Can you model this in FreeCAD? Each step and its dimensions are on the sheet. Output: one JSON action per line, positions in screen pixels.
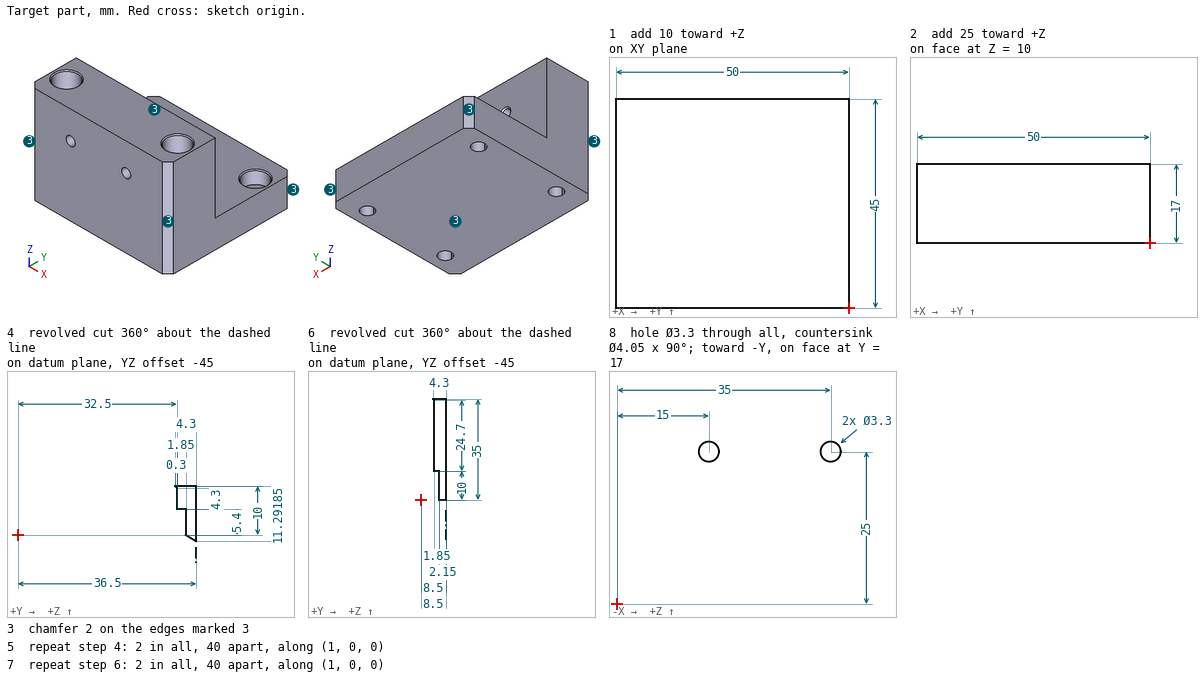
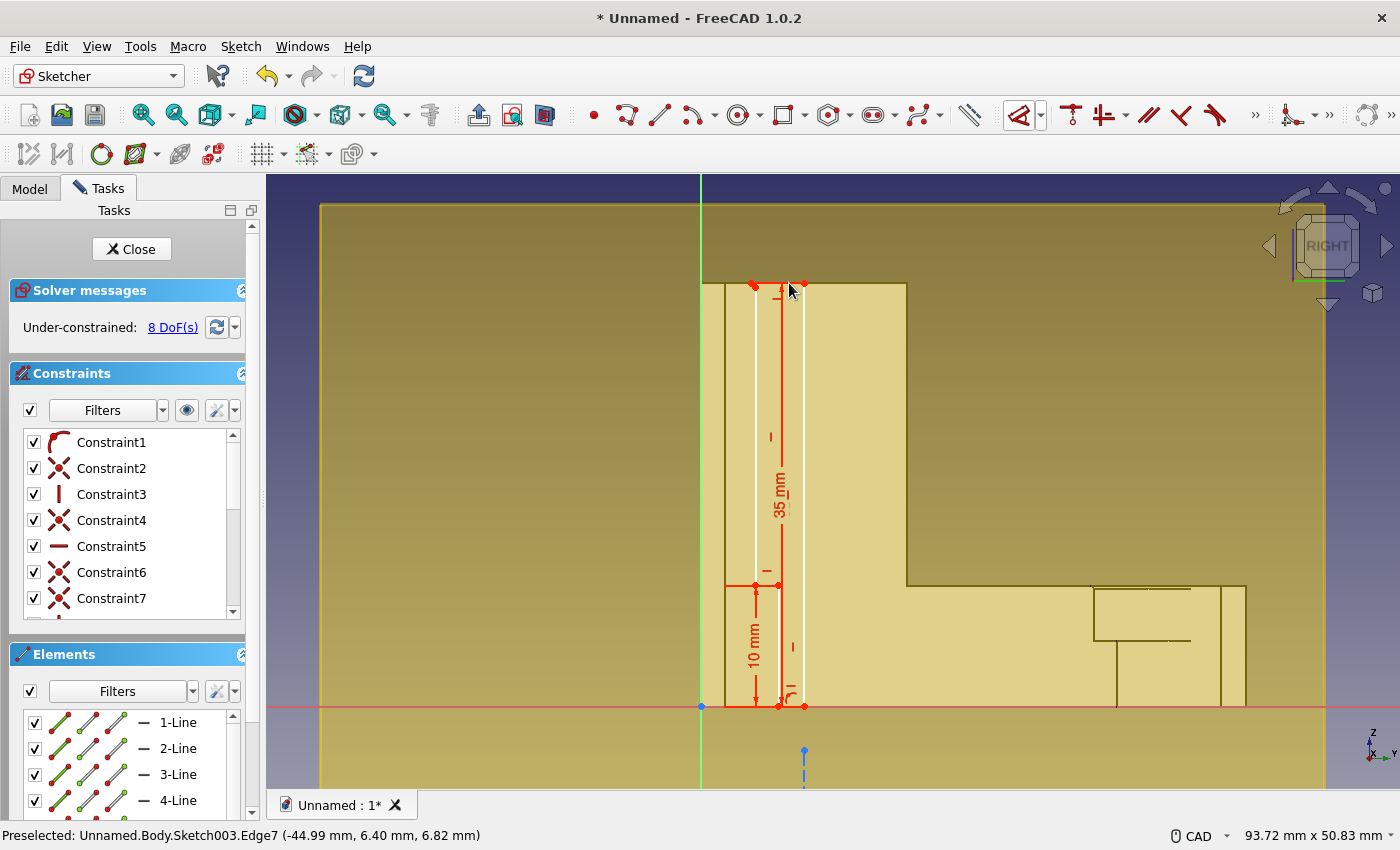
{"action": "left_click", "coordinate": [788, 283]}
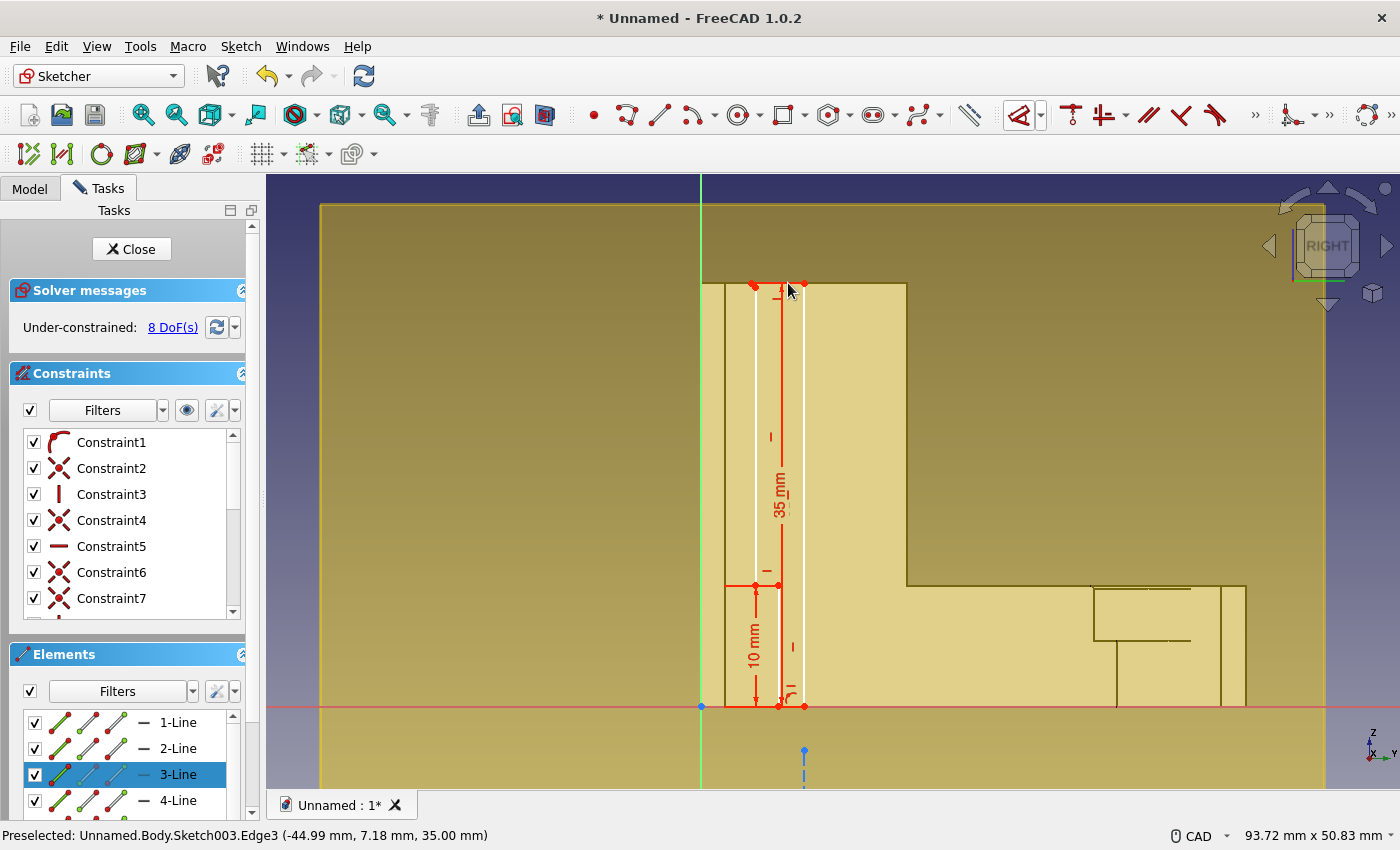
{"action": "key", "text": "l"}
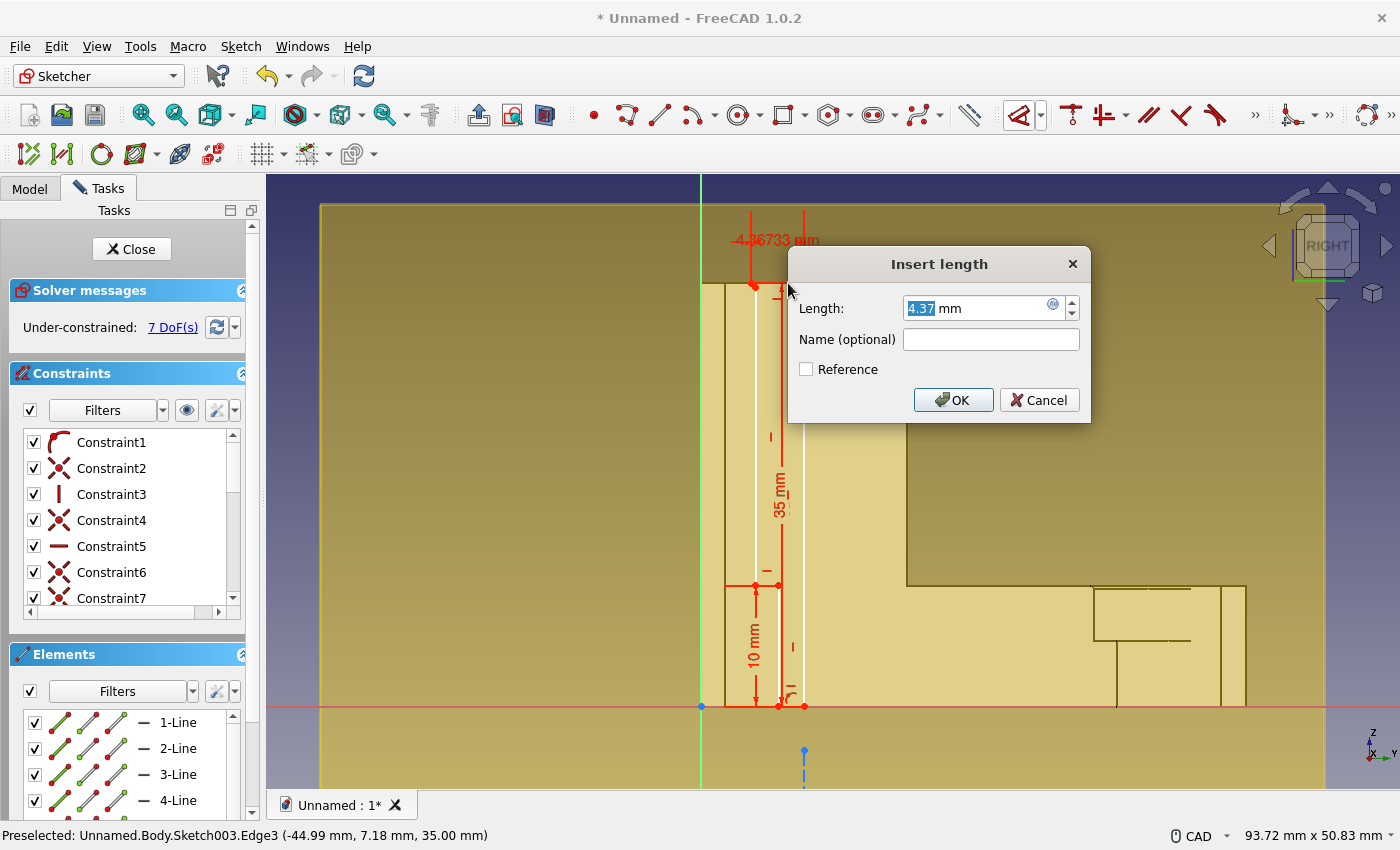
{"action": "type", "text": "4.3"}
{"action": "key", "text": "Return"}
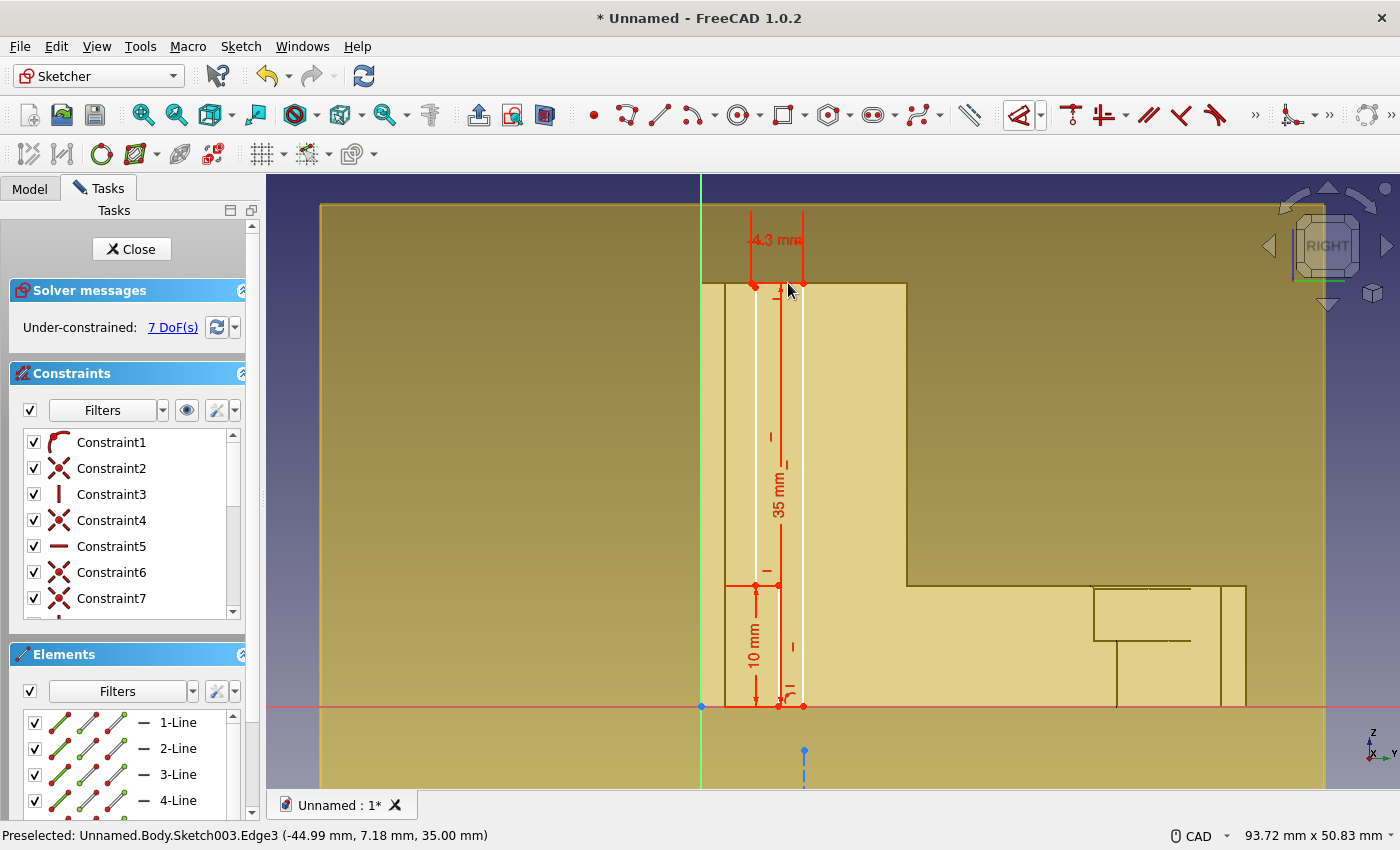
{"action": "scroll", "coordinate": [788, 707], "scroll_direction": "up", "scroll_amount": 3}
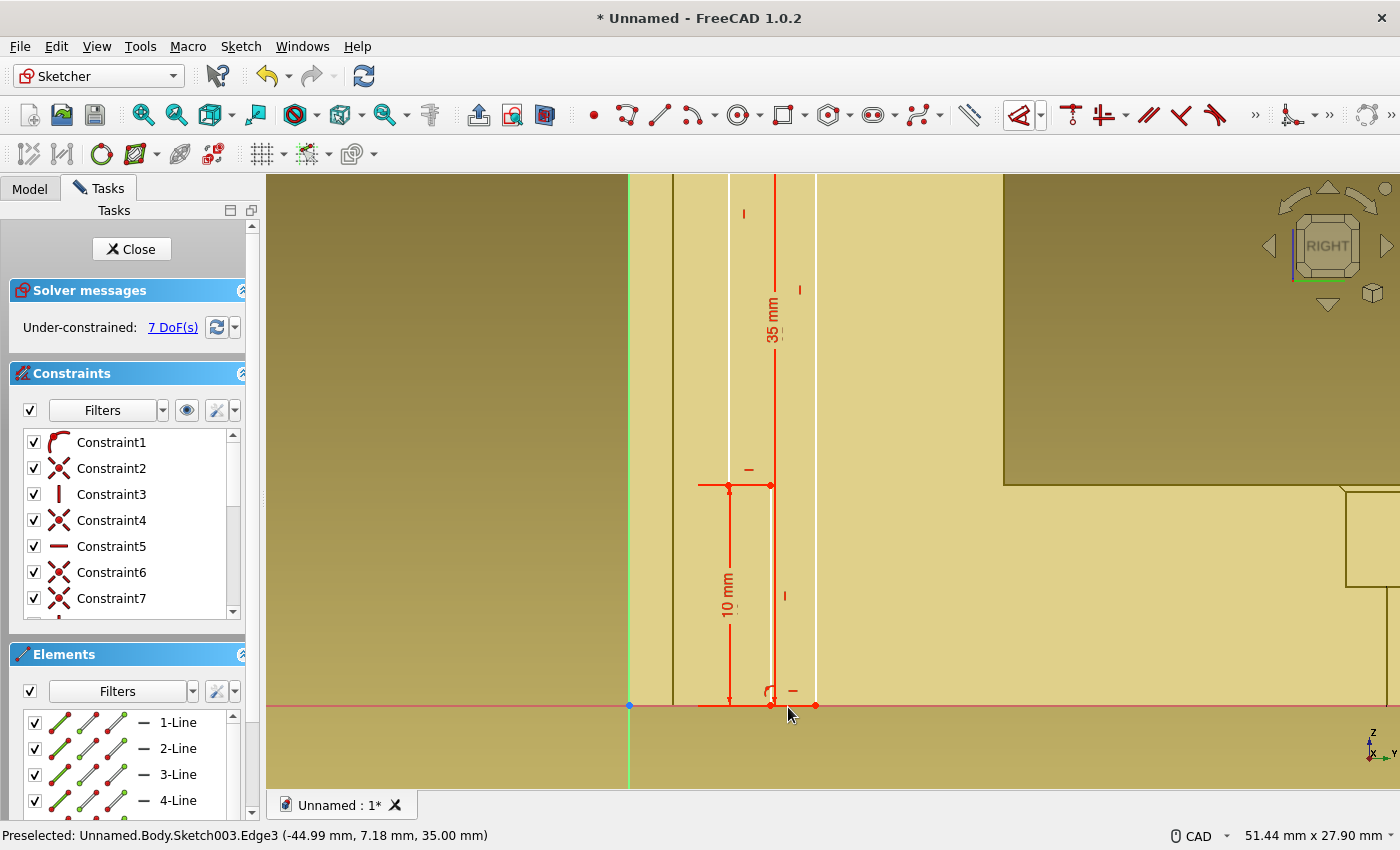
{"action": "left_click", "coordinate": [789, 706]}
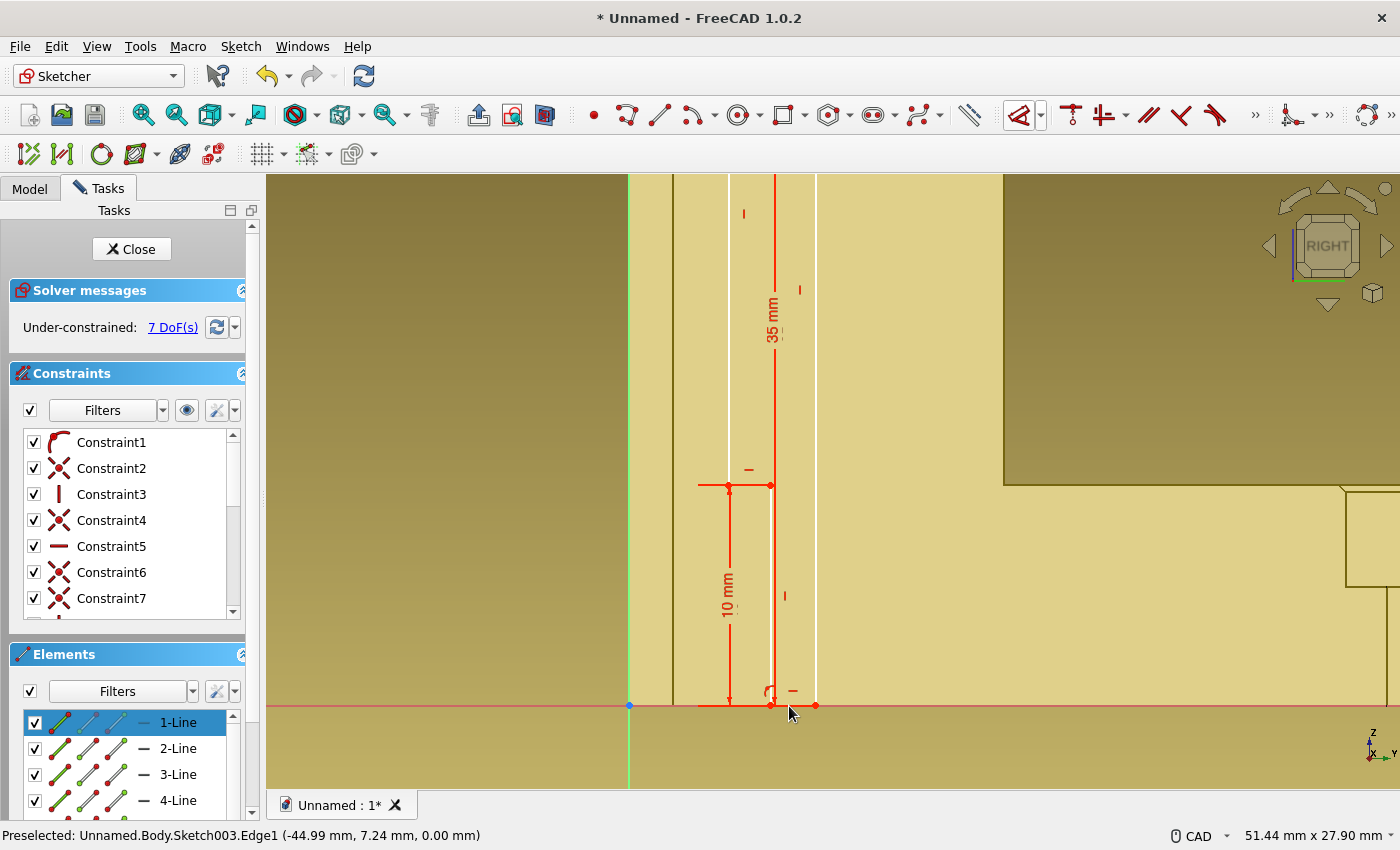
{"action": "key", "text": "l"}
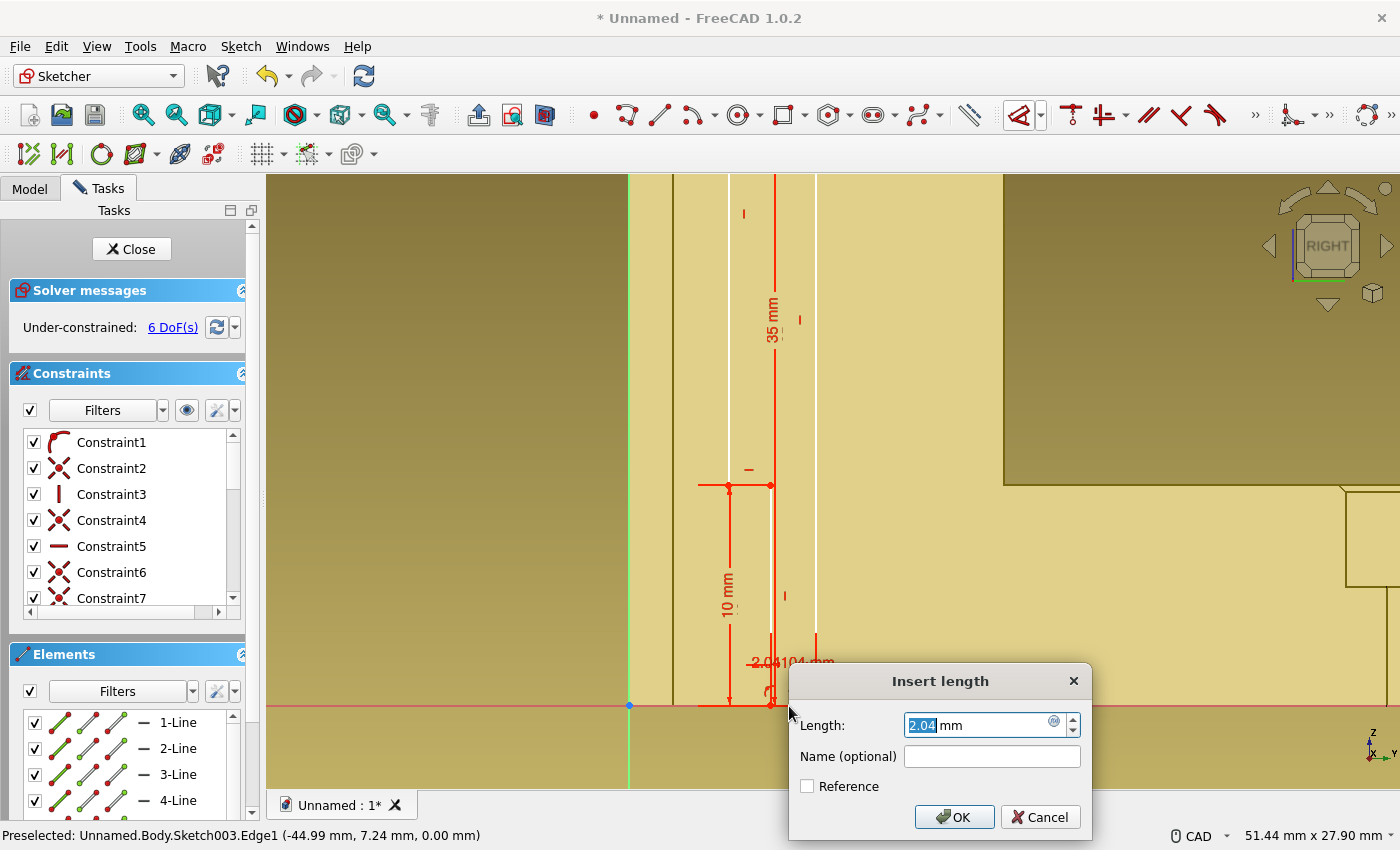
{"action": "type", "text": "2.15"}
{"action": "key", "text": "Return"}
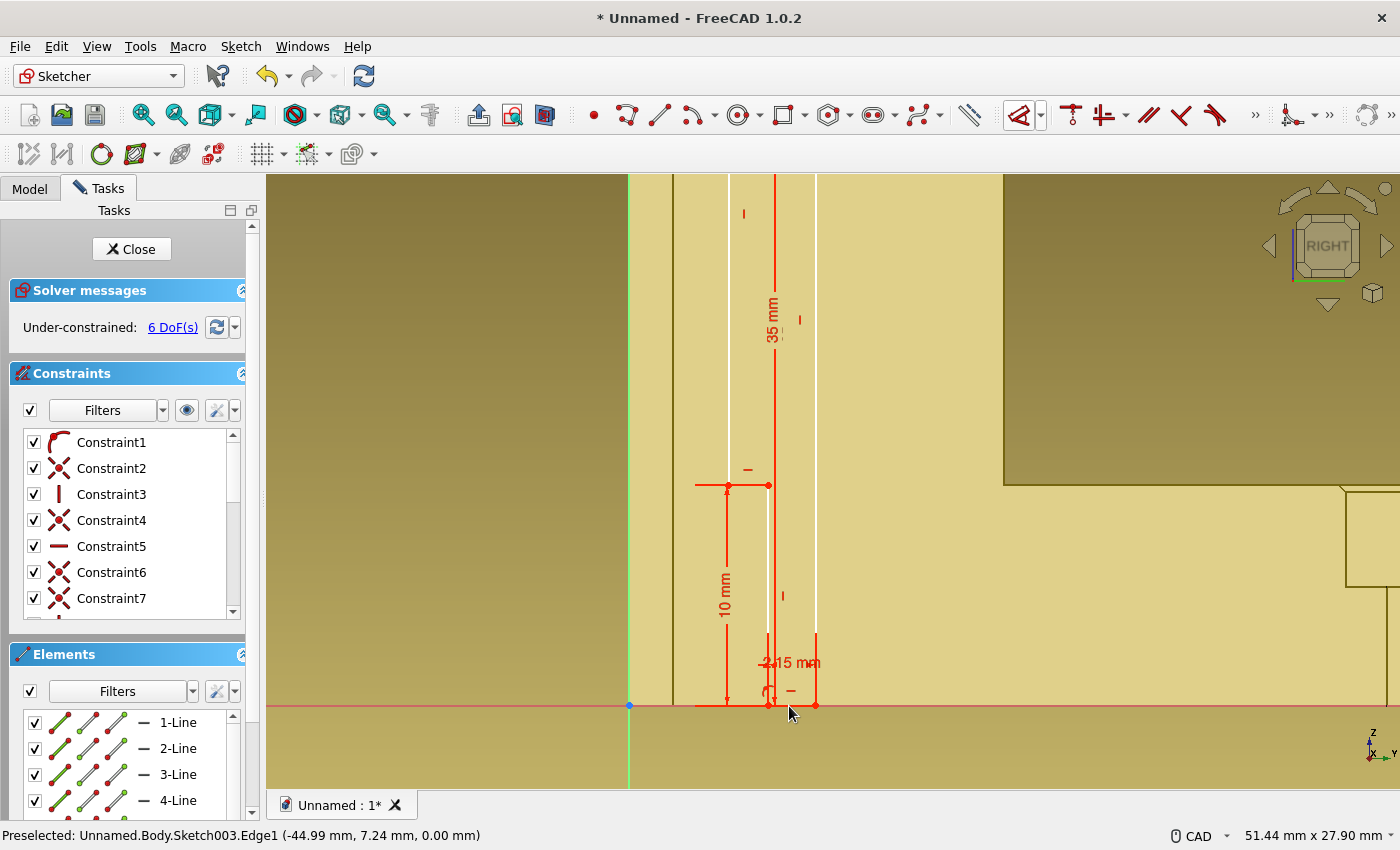
{"action": "left_click", "coordinate": [729, 322]}